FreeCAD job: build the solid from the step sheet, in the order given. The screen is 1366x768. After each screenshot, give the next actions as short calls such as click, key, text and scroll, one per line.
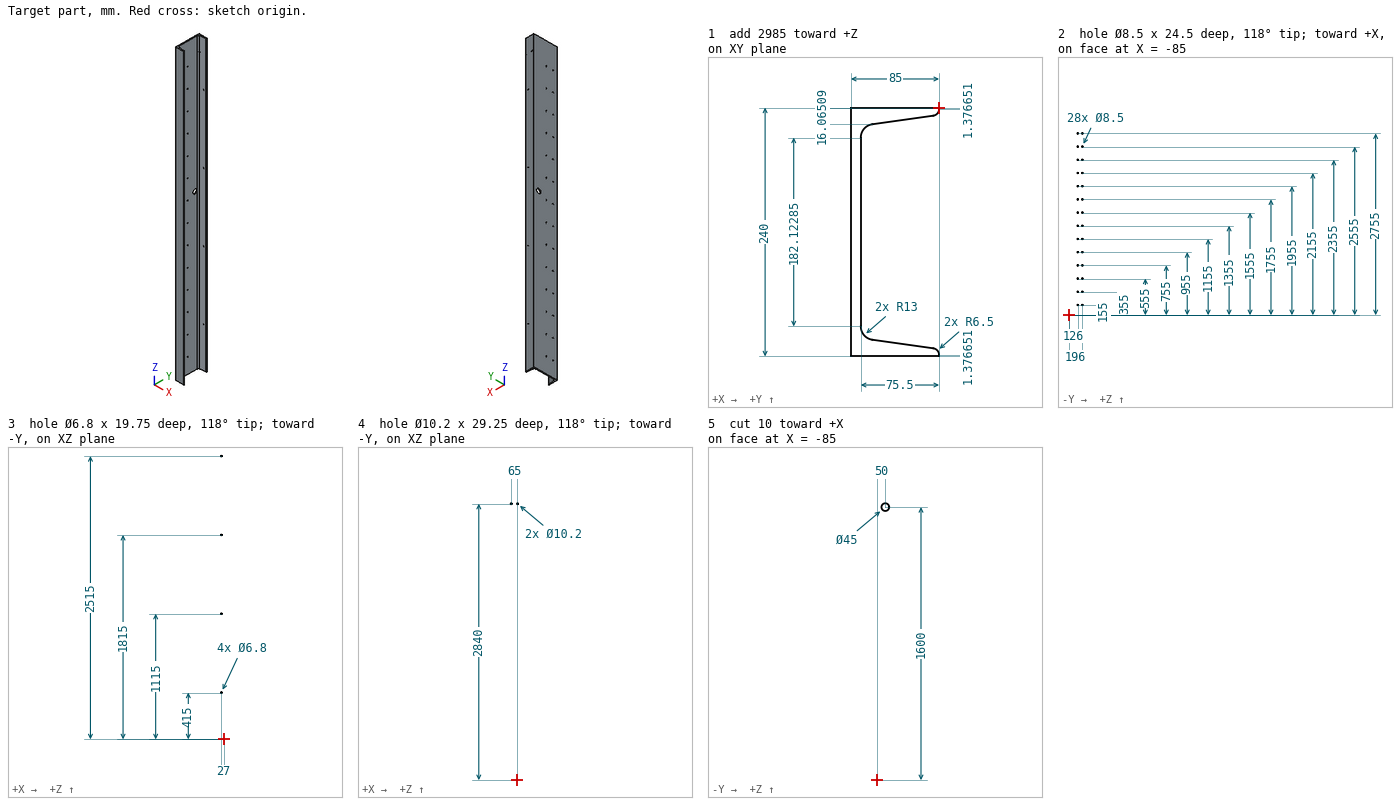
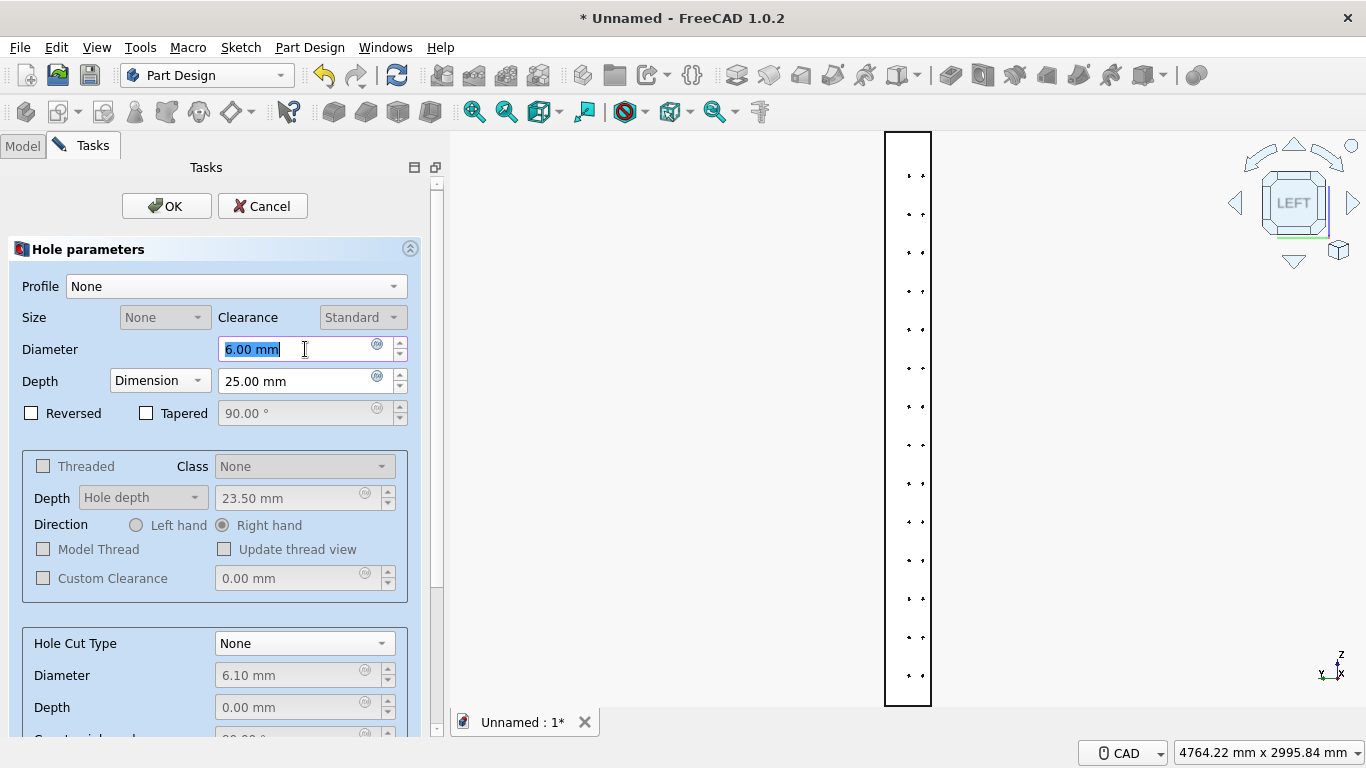
text(10.2)
key(Tab)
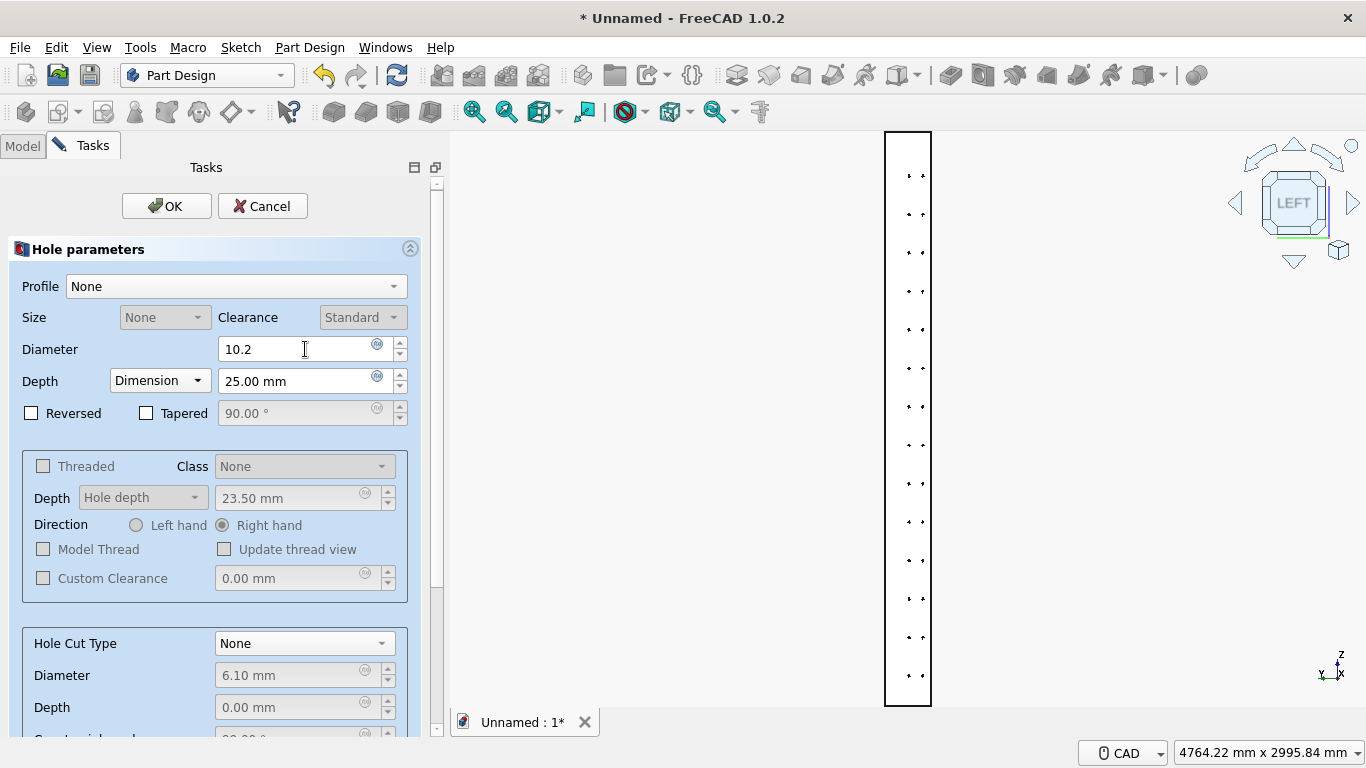
triple_click(305, 381)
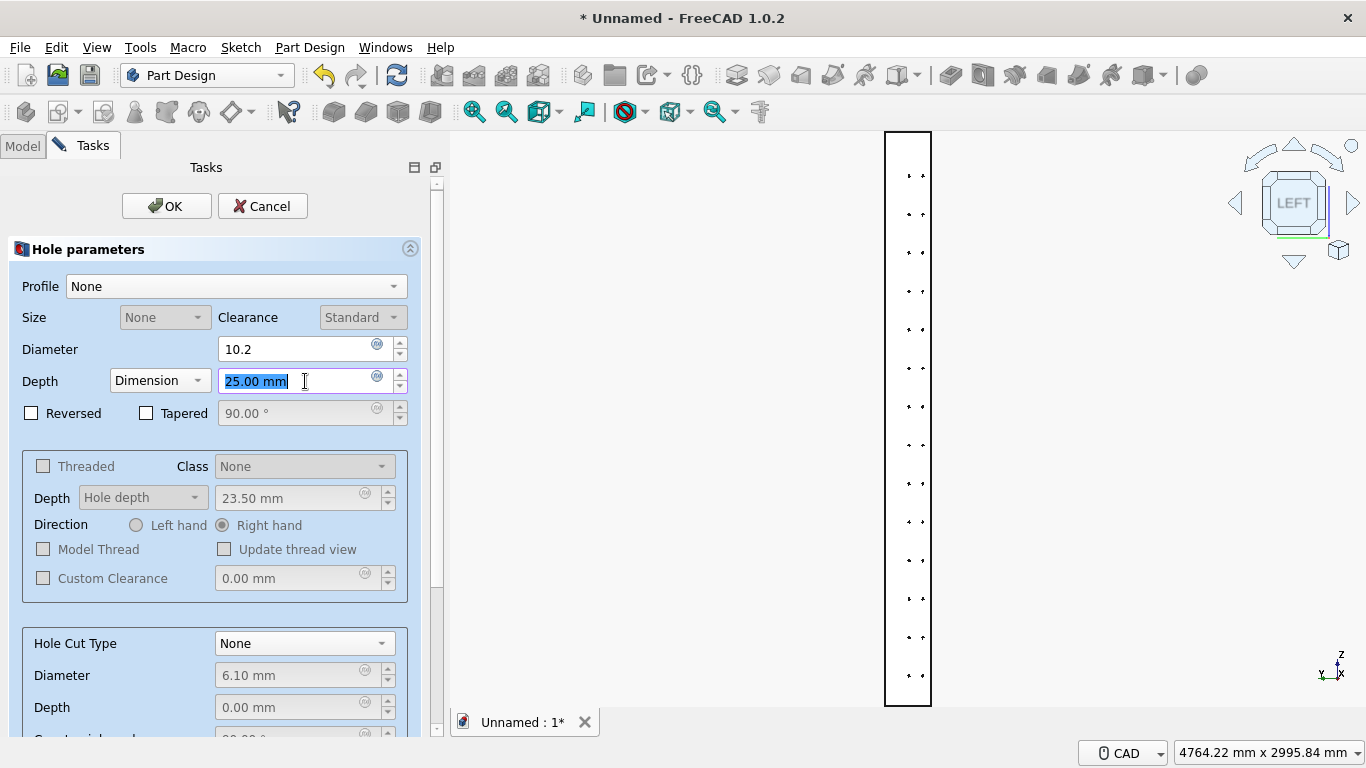
text(29.25)
key(Tab)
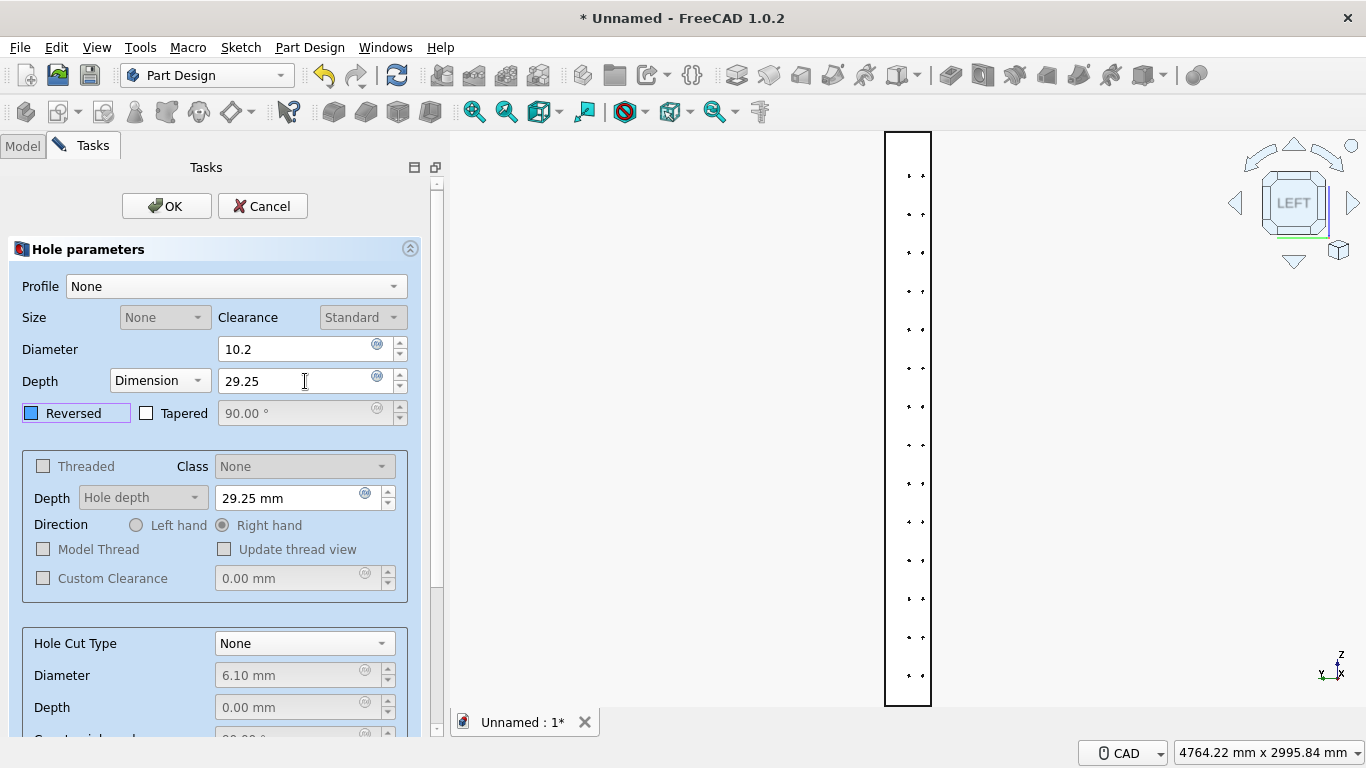
click(30, 413)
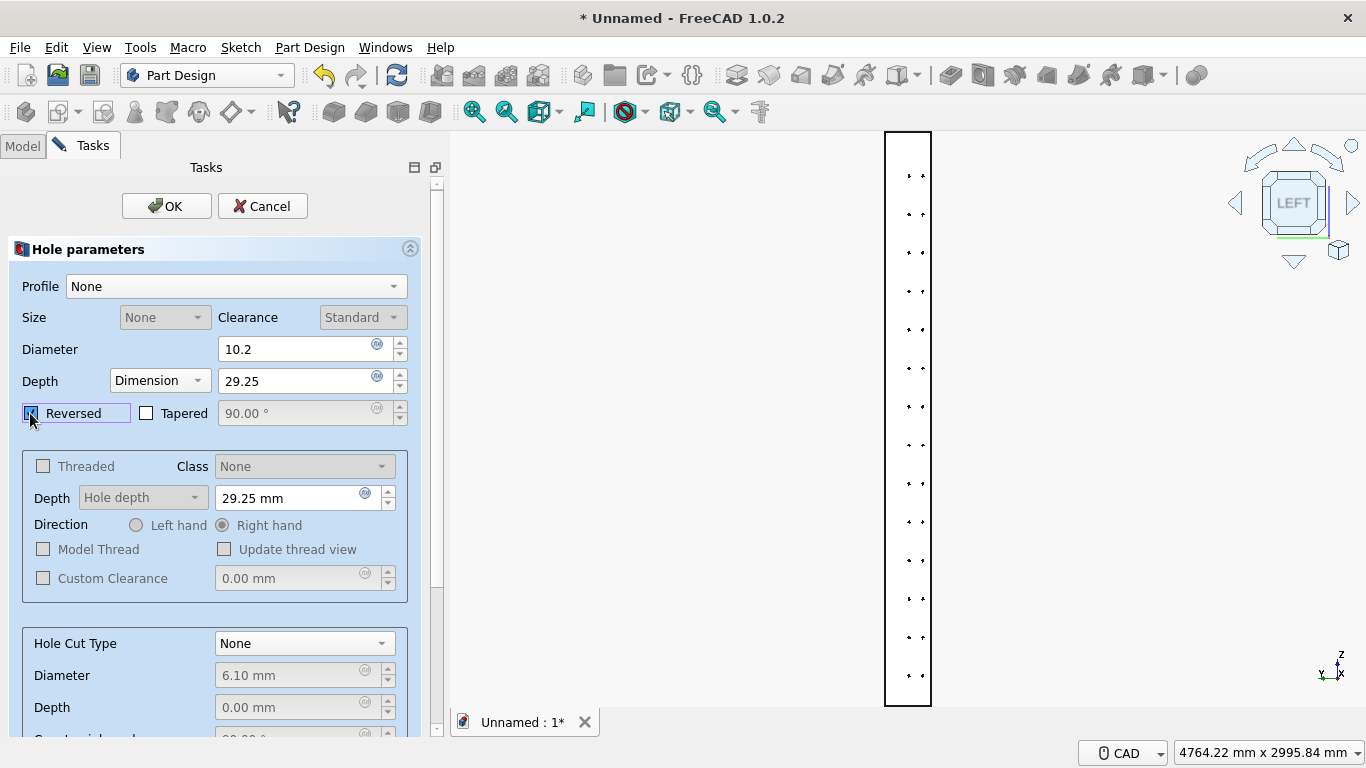
click(167, 206)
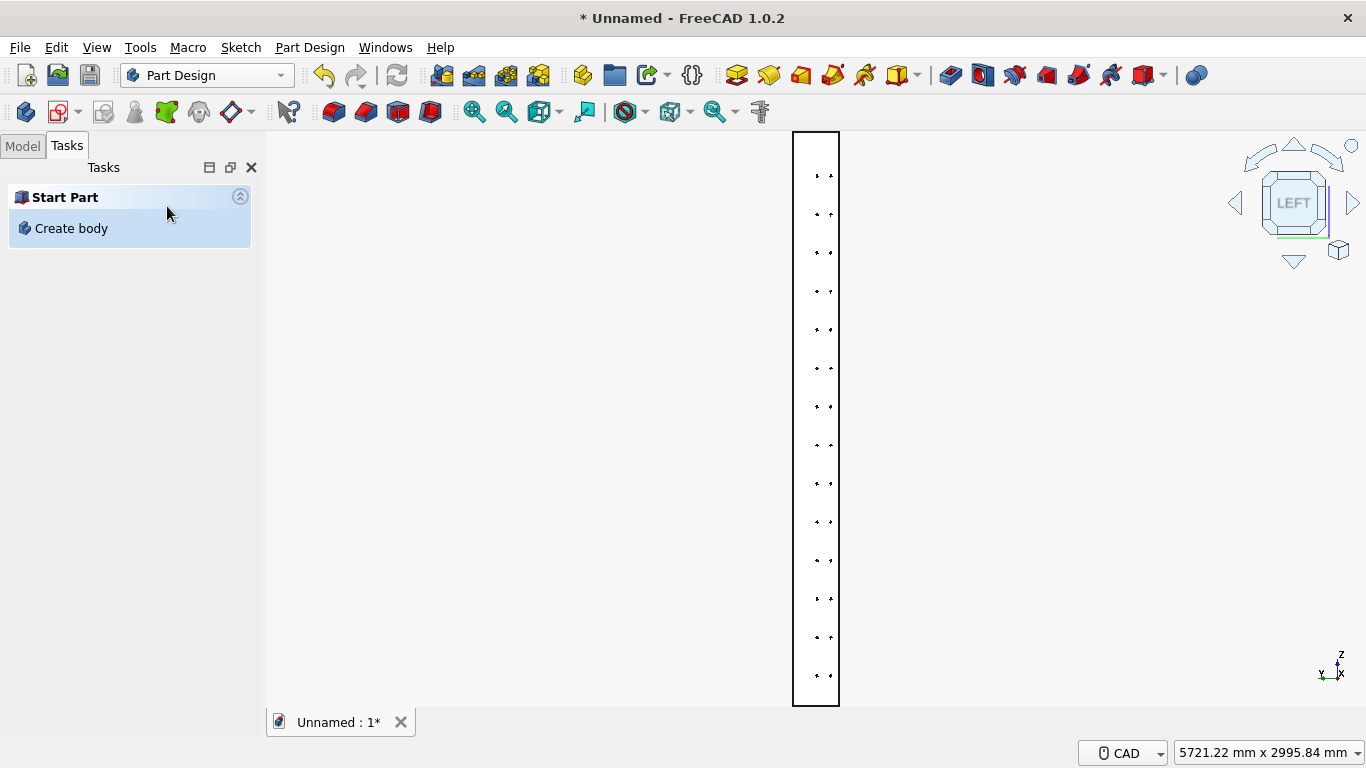
click(823, 500)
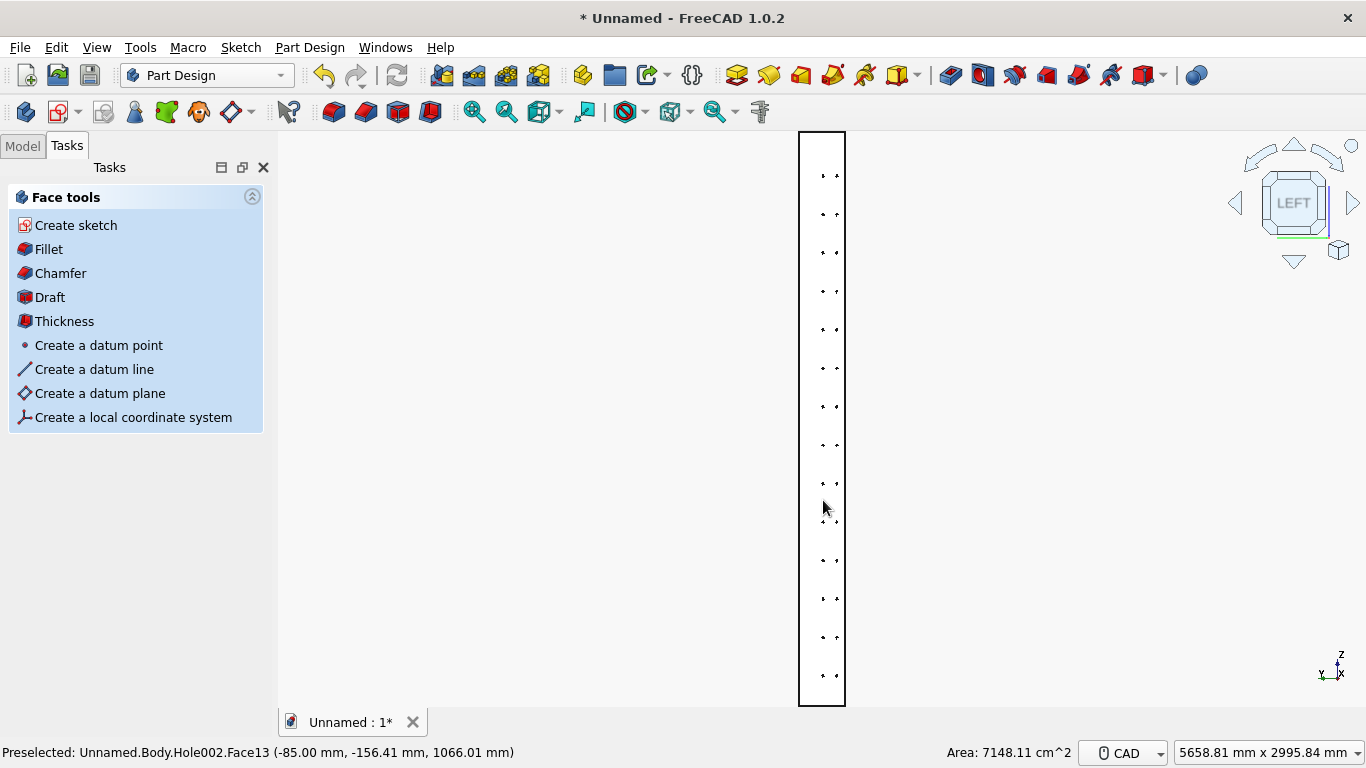
click(58, 112)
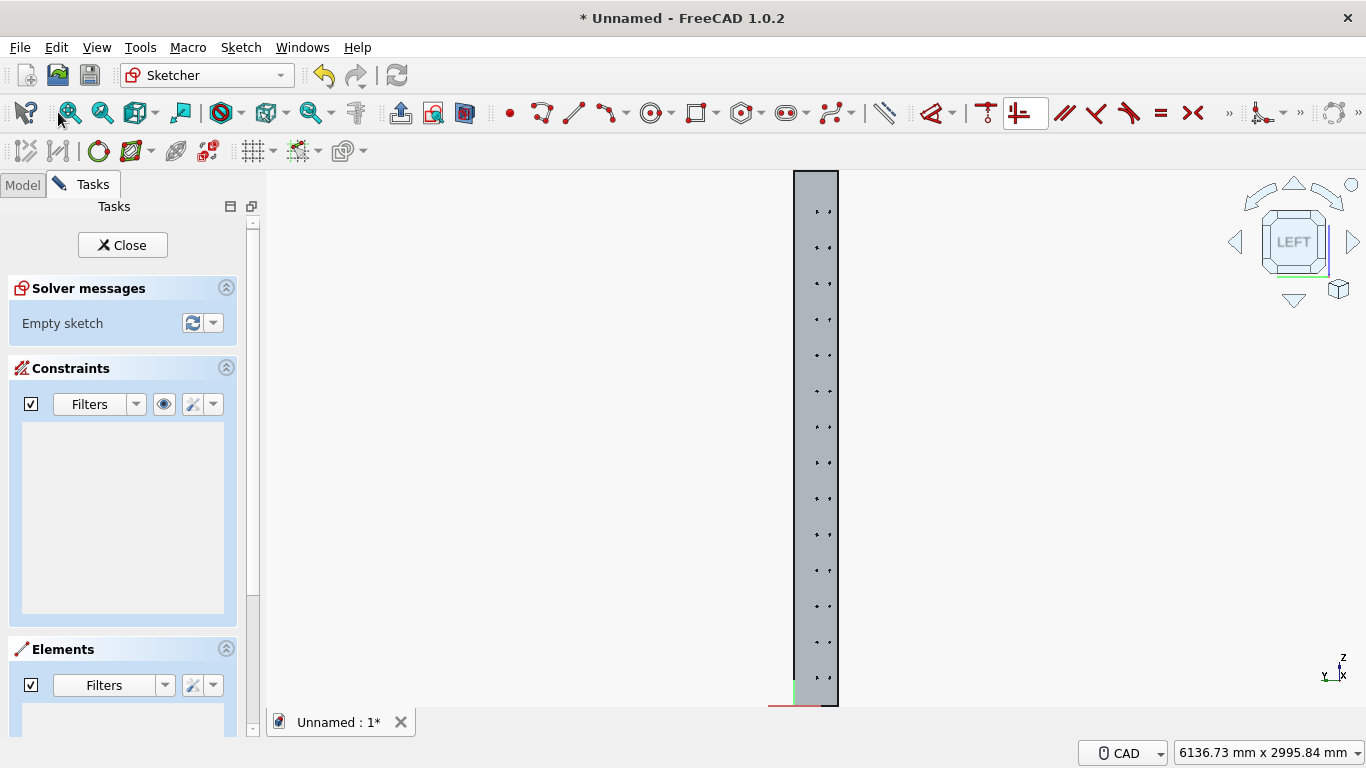
scroll(806, 418, up, 15)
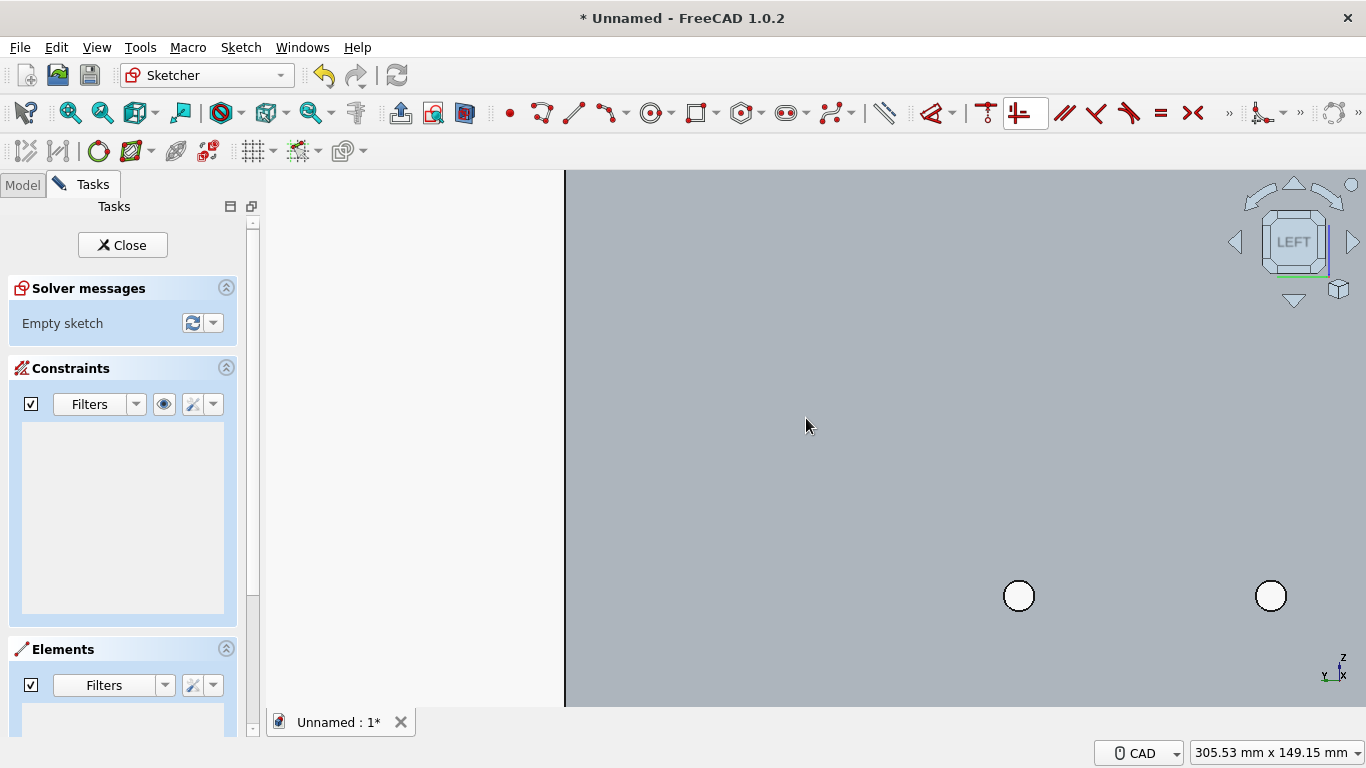
scroll(744, 430, up, 4)